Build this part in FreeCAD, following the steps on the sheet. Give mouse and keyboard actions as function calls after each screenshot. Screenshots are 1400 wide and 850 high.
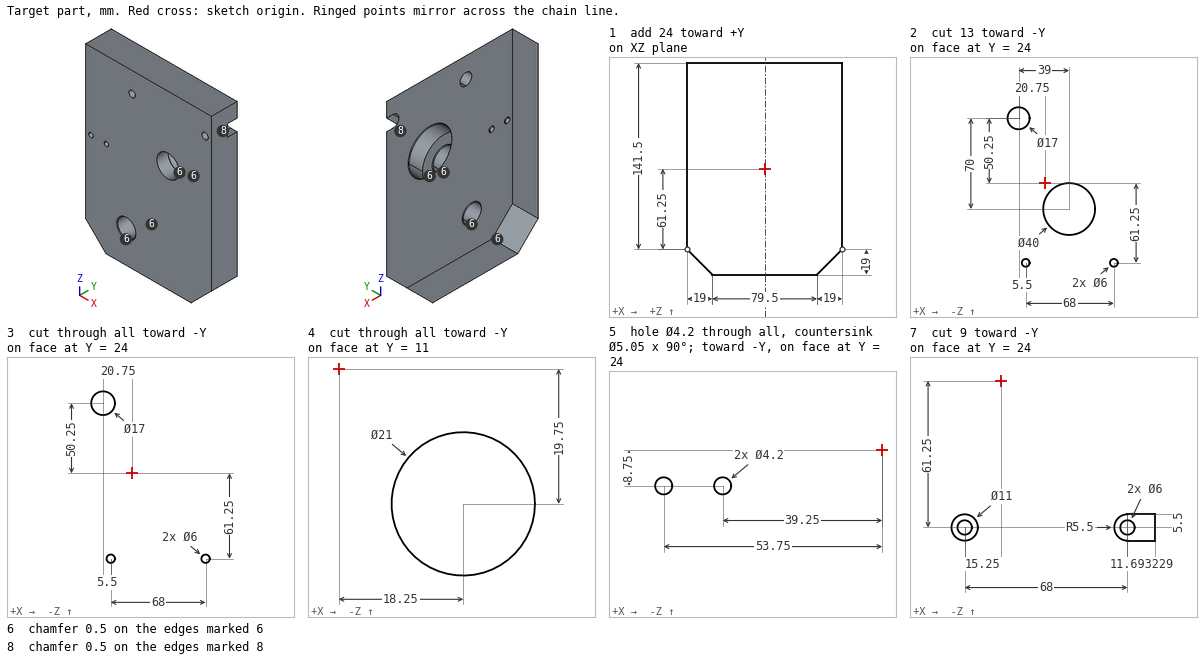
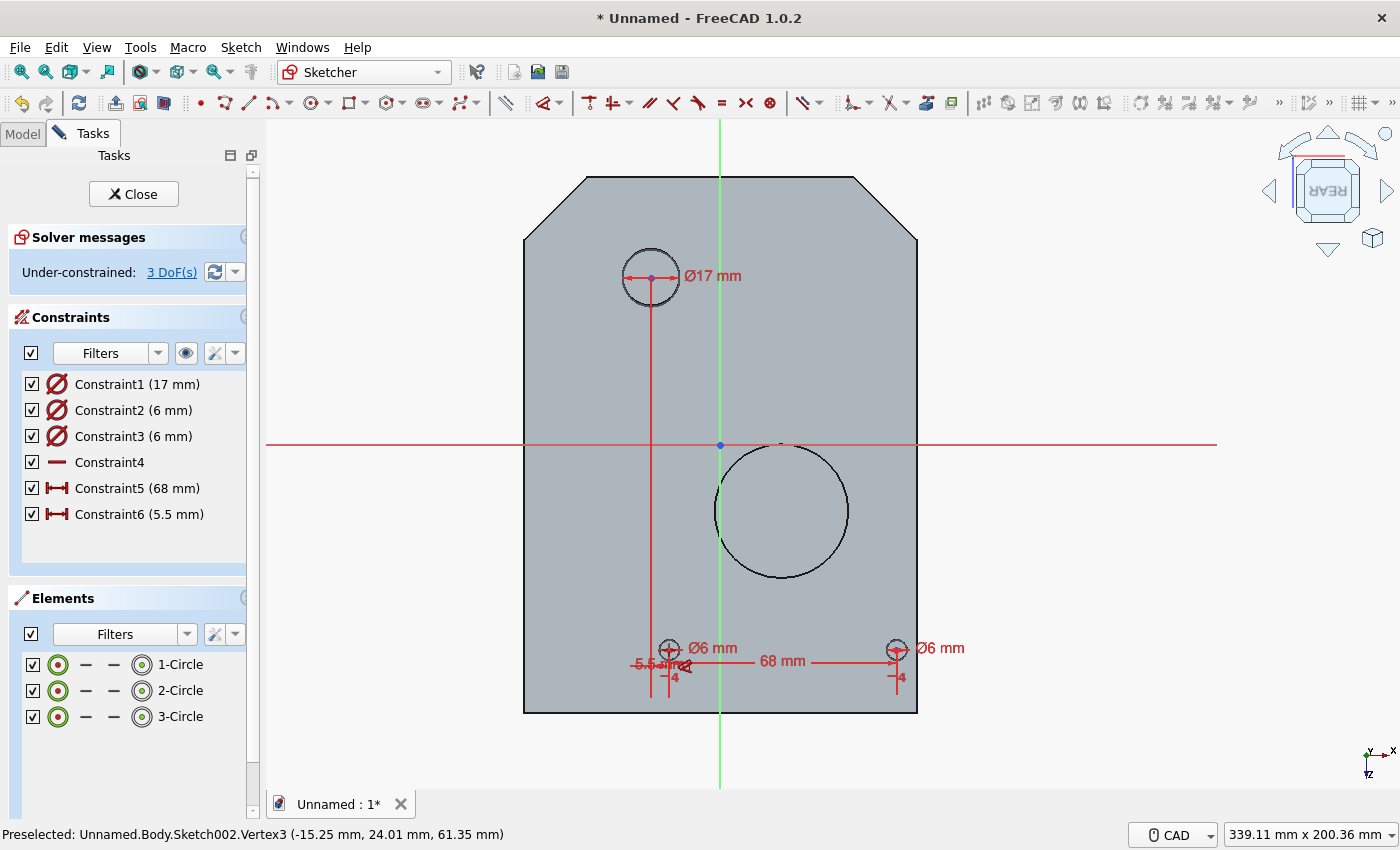
click(651, 278)
click(686, 244)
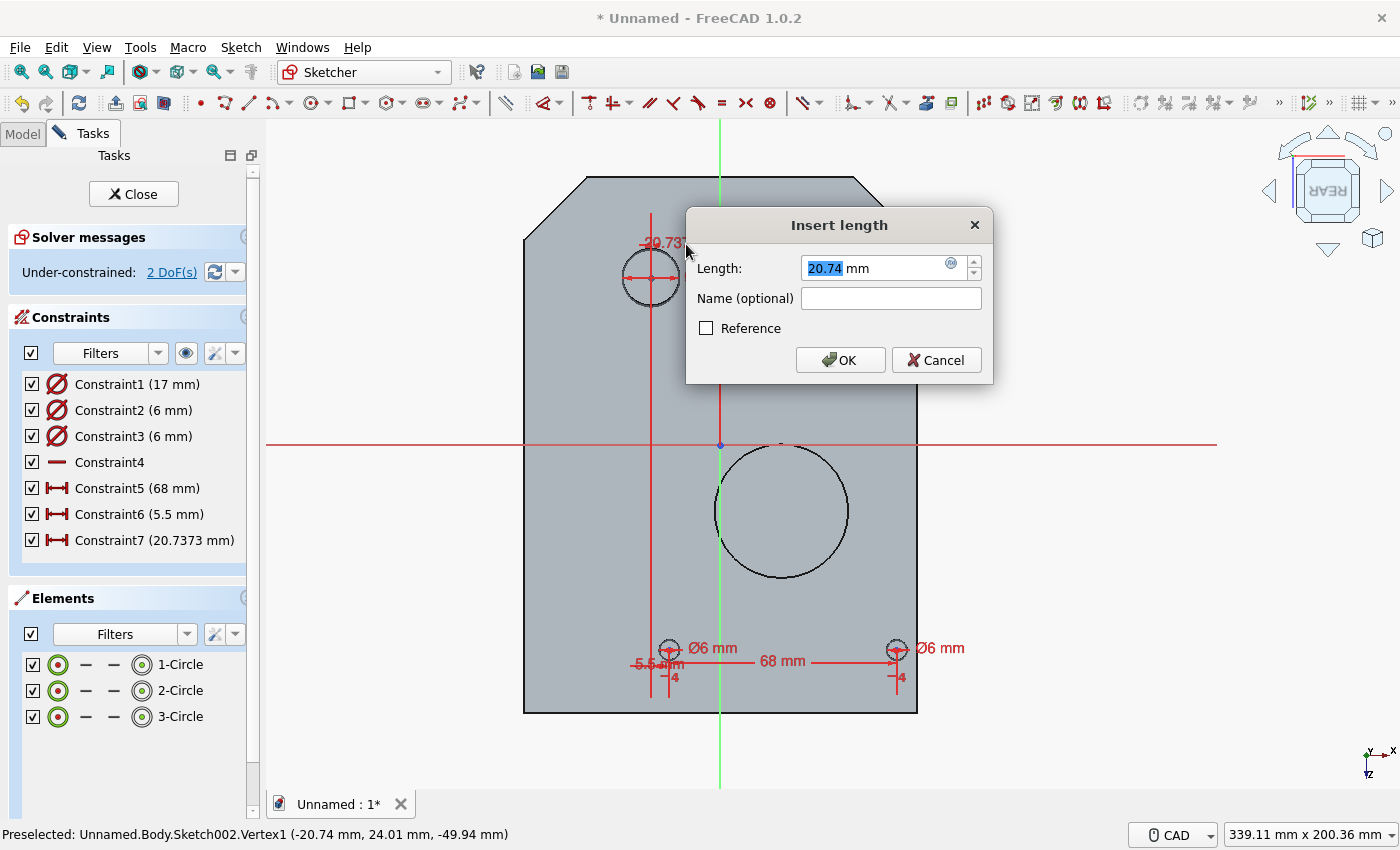
text(20.75)
key(Return)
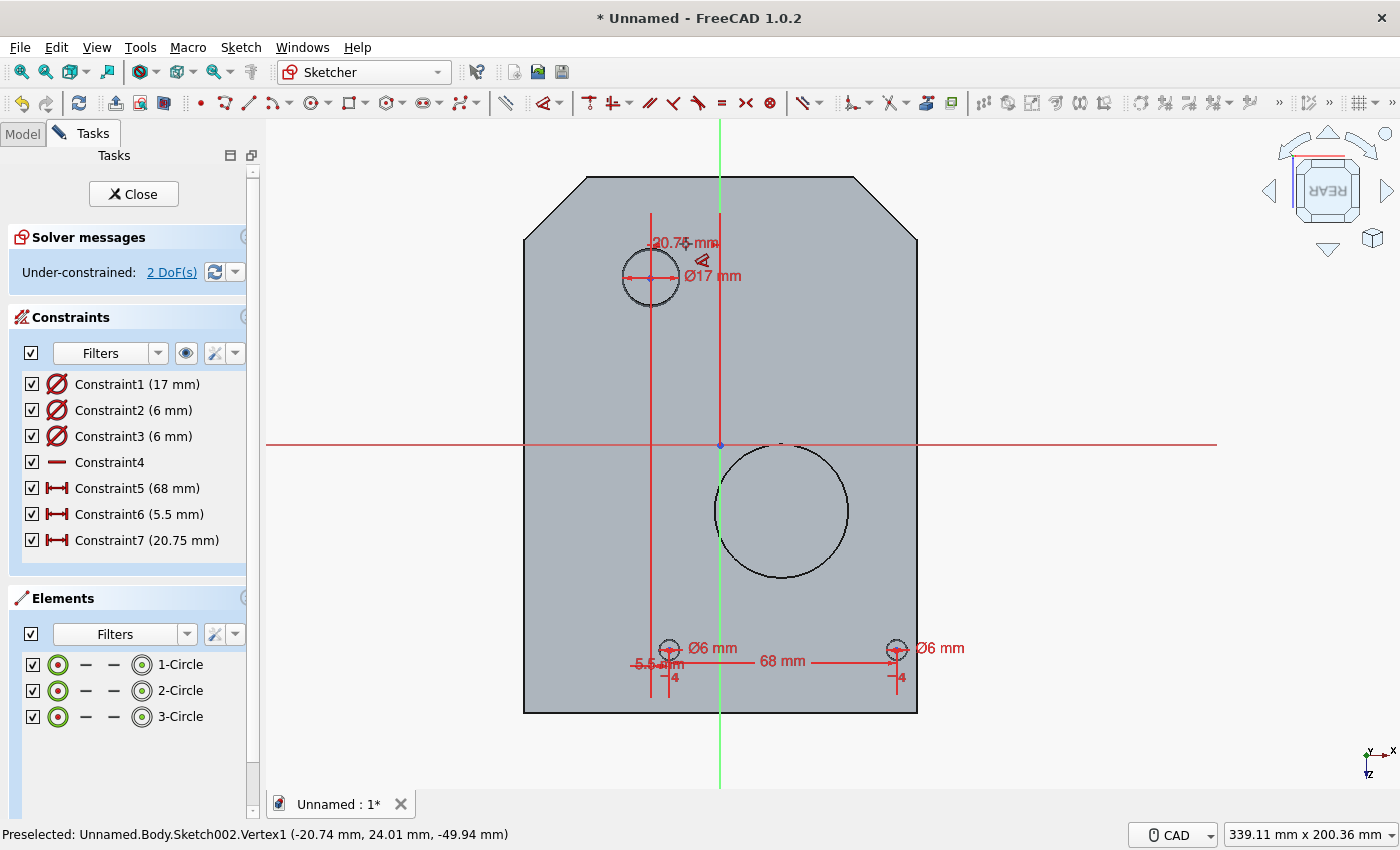
click(651, 278)
click(617, 362)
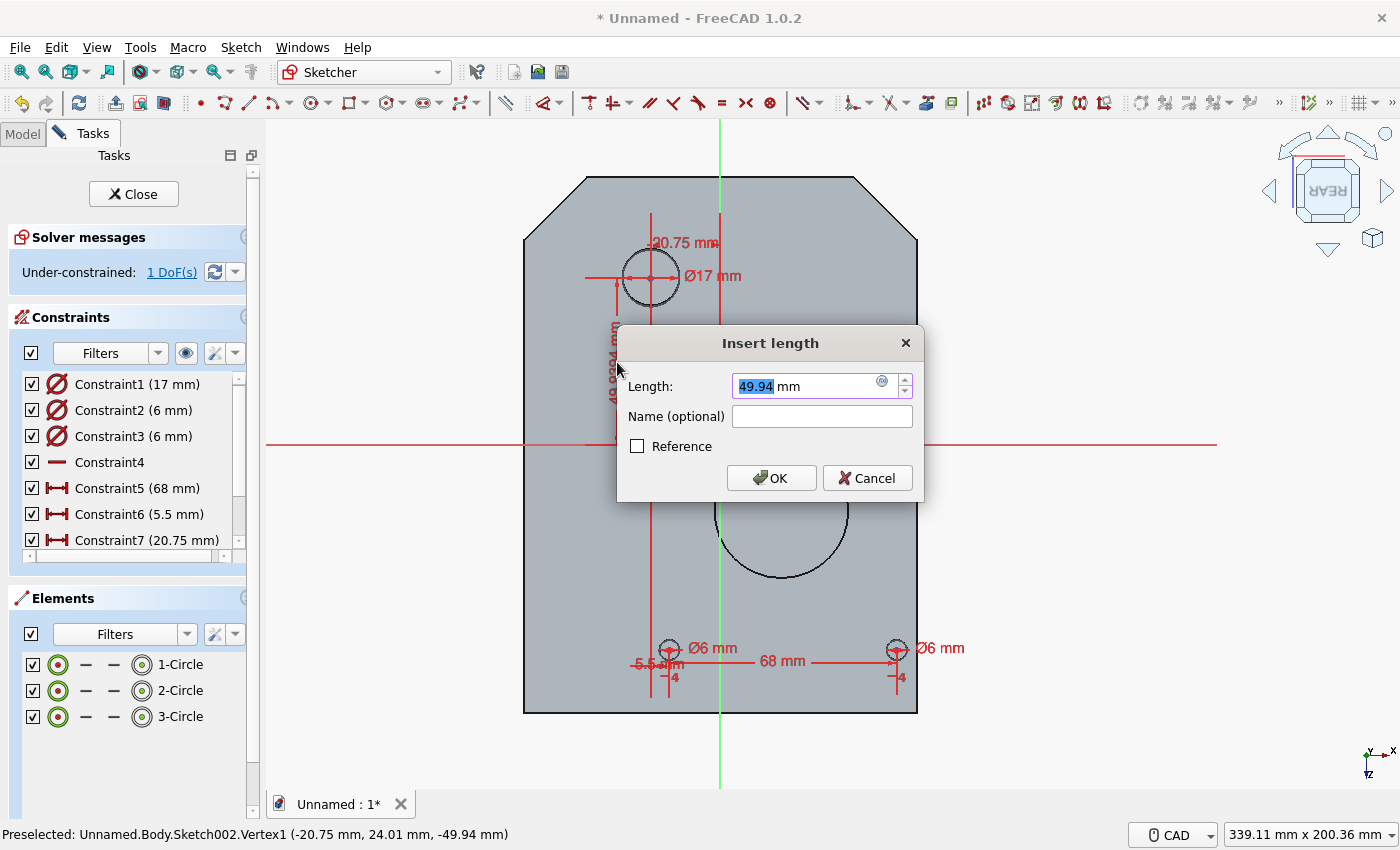
text(50.25)
key(Return)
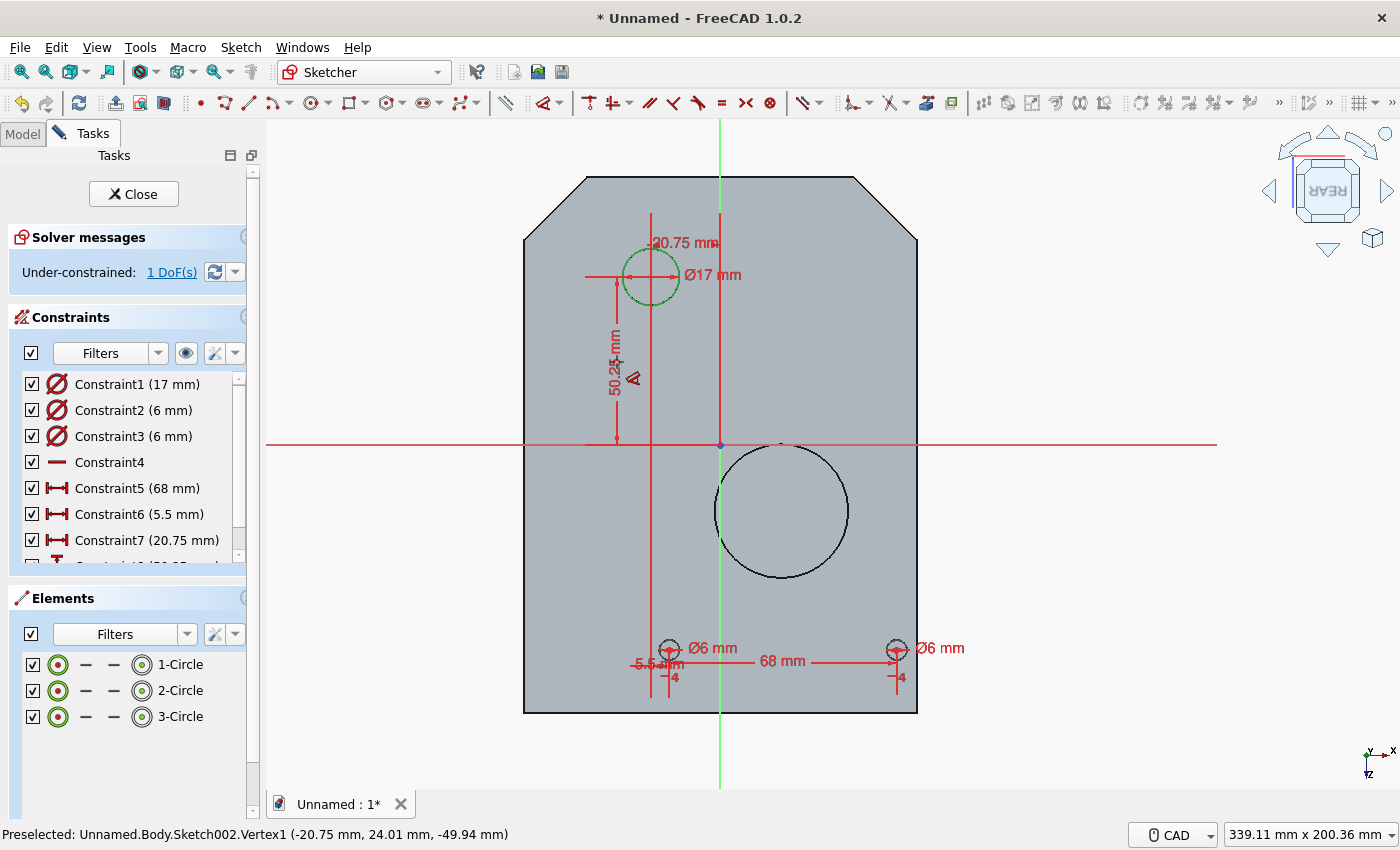
click(897, 650)
click(931, 548)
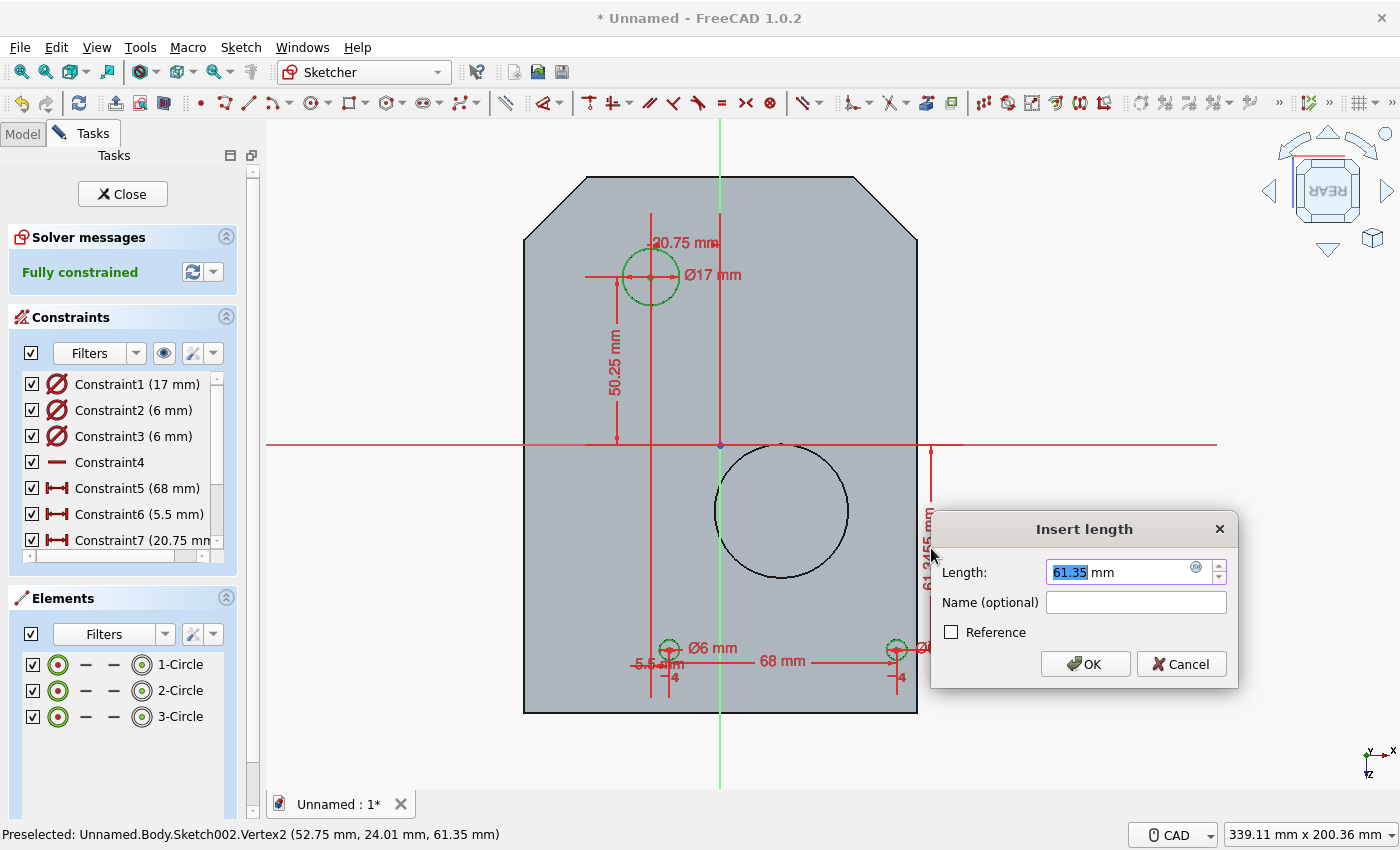
text(61.25)
key(Return)
key(Escape)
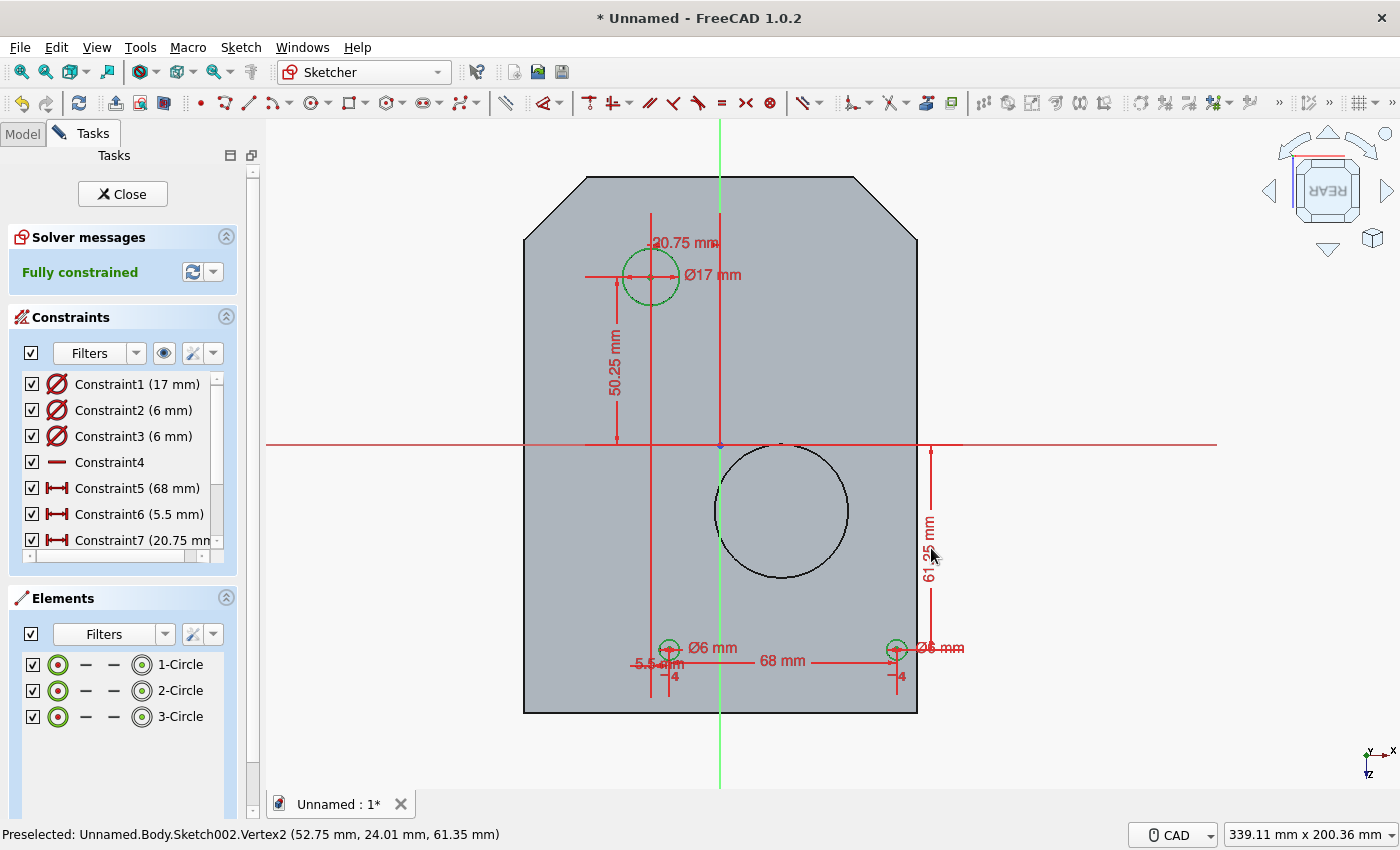
click(123, 194)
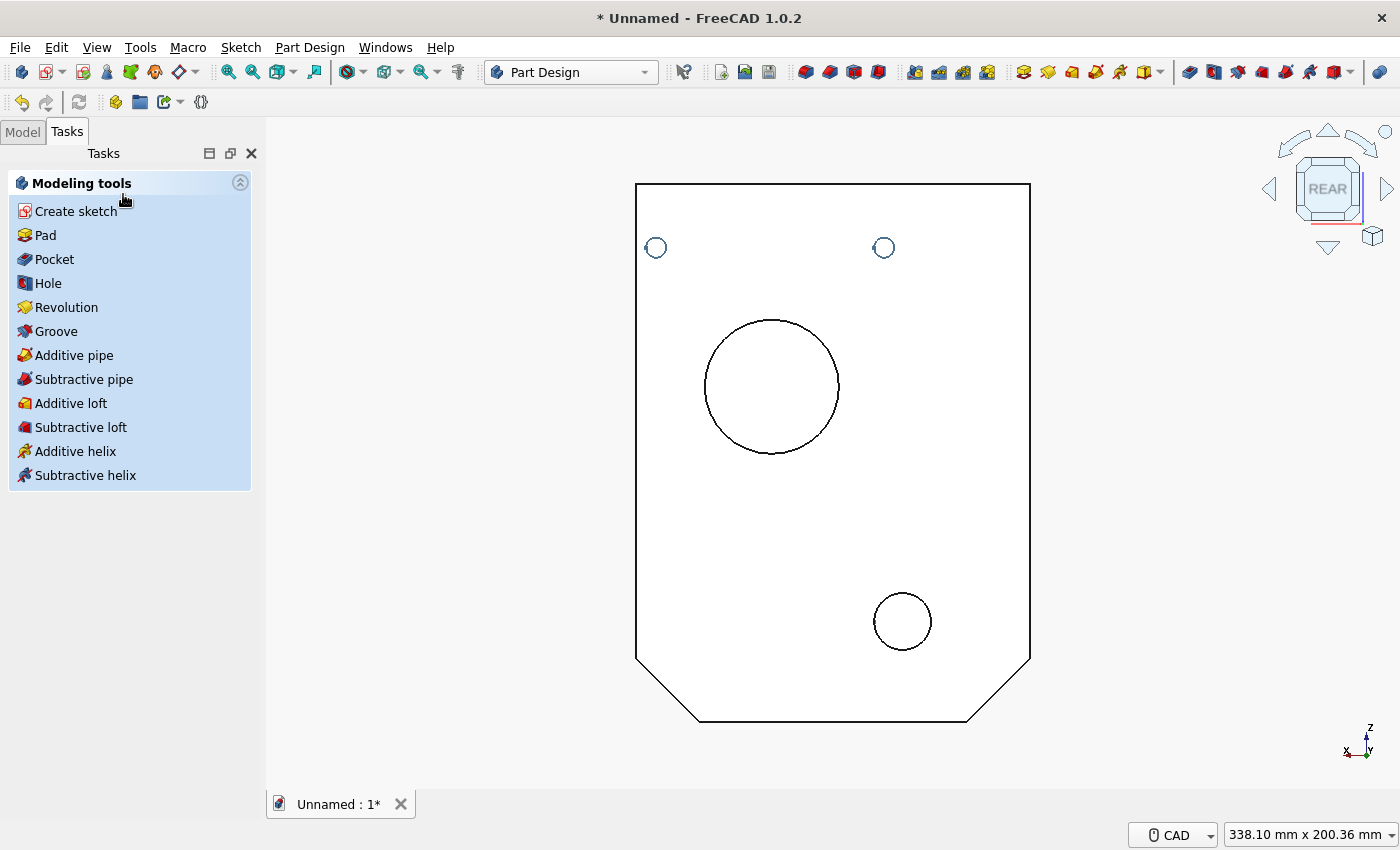
click(1190, 72)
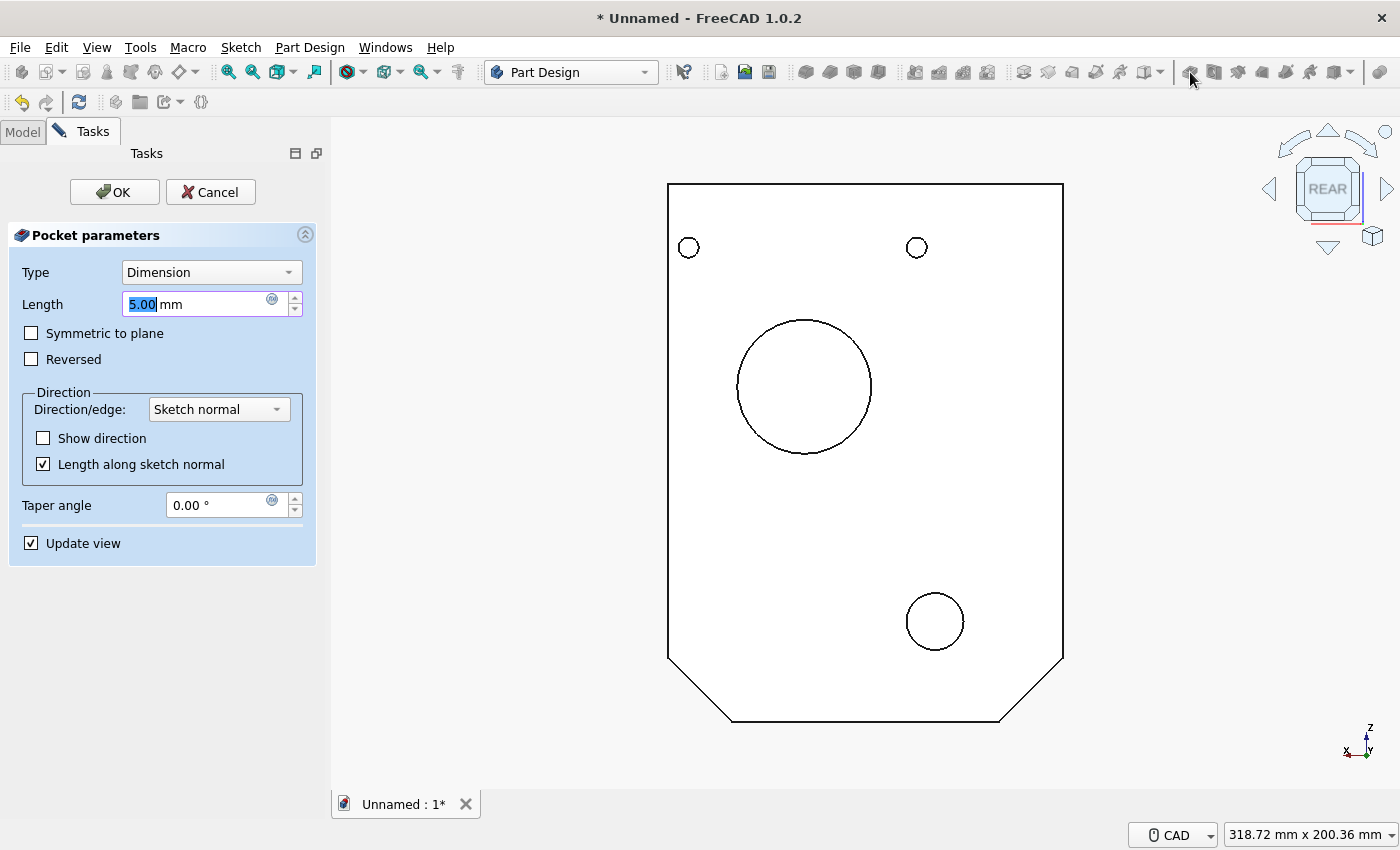
click(212, 272)